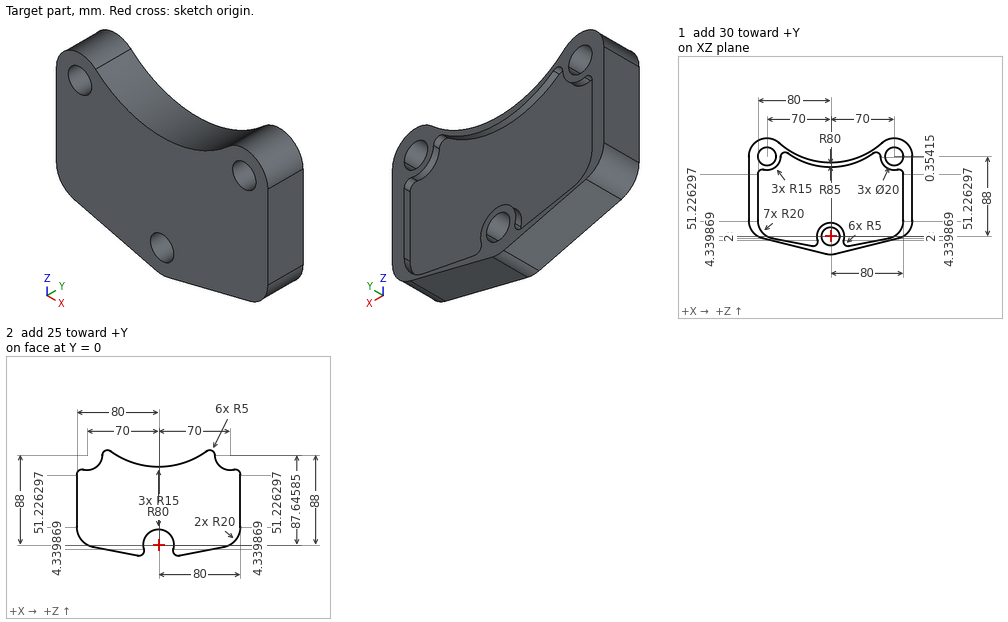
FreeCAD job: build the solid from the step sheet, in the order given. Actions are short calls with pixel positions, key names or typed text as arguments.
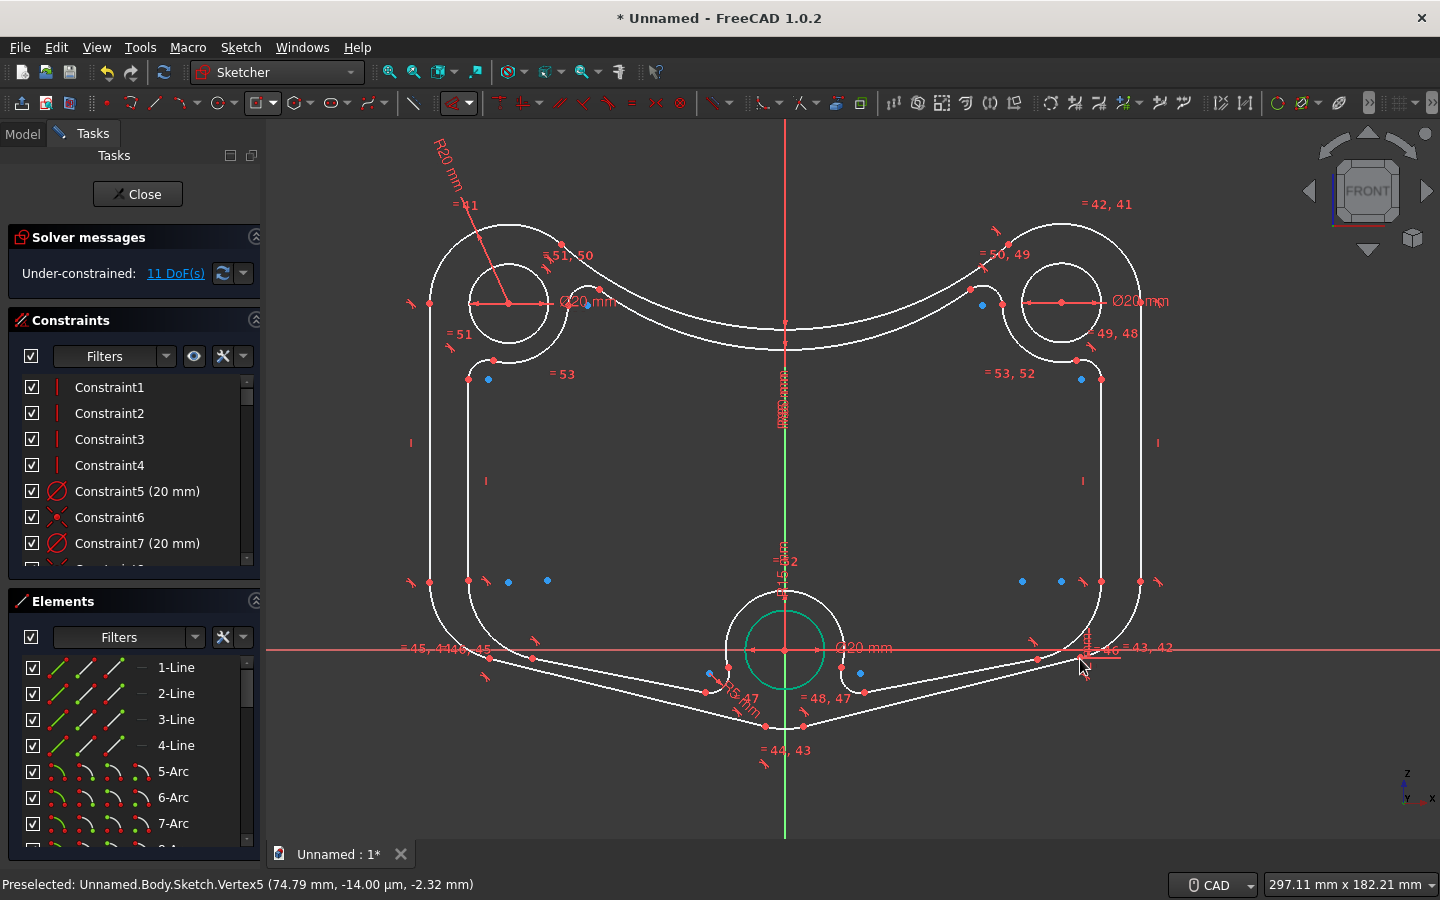
scroll(490, 659, up, 9)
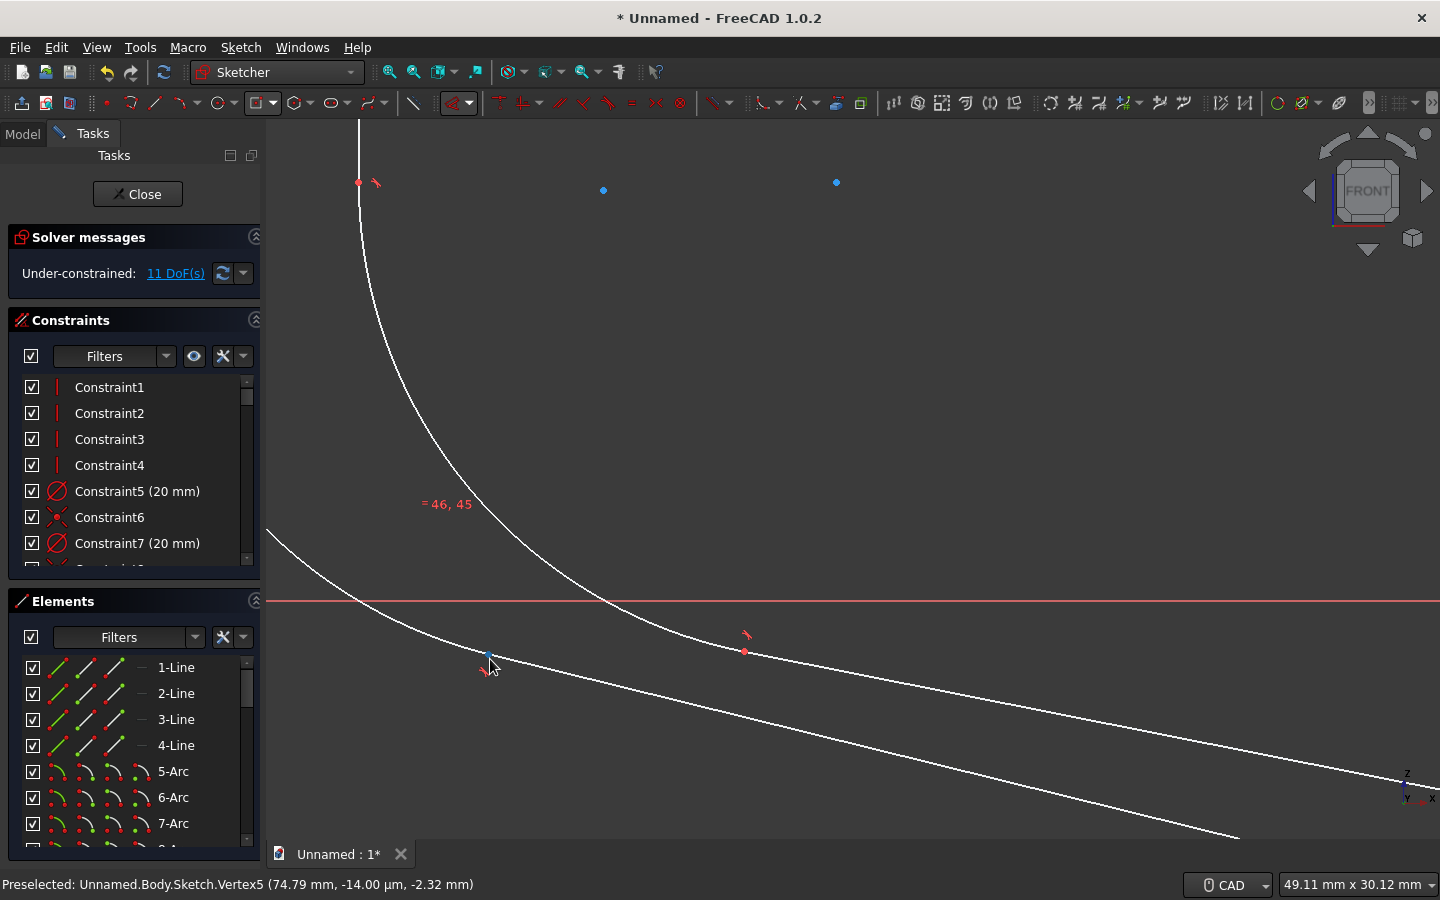
click(489, 654)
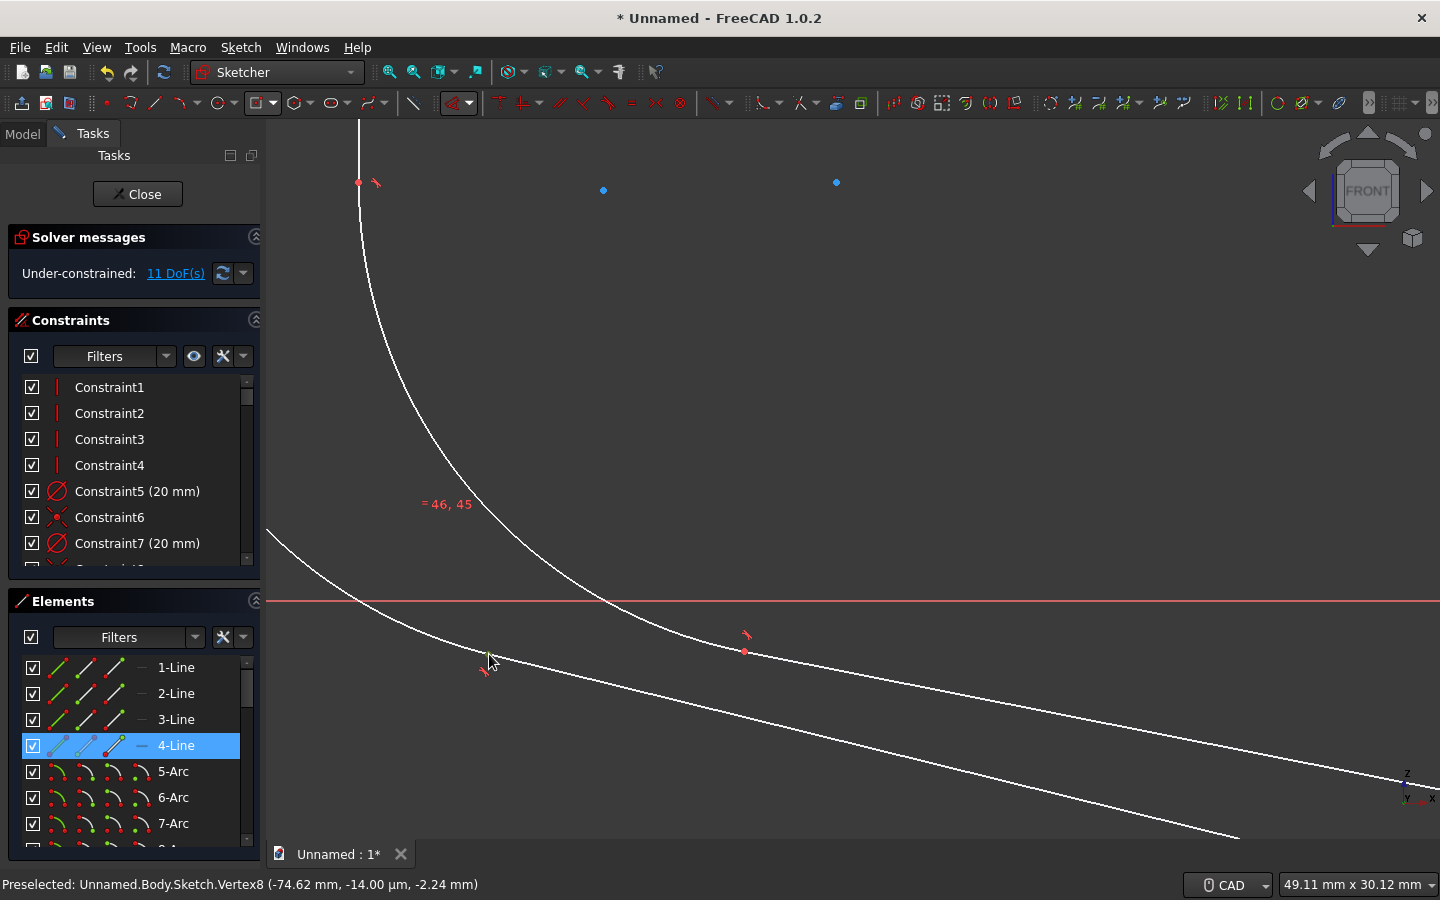
key(i)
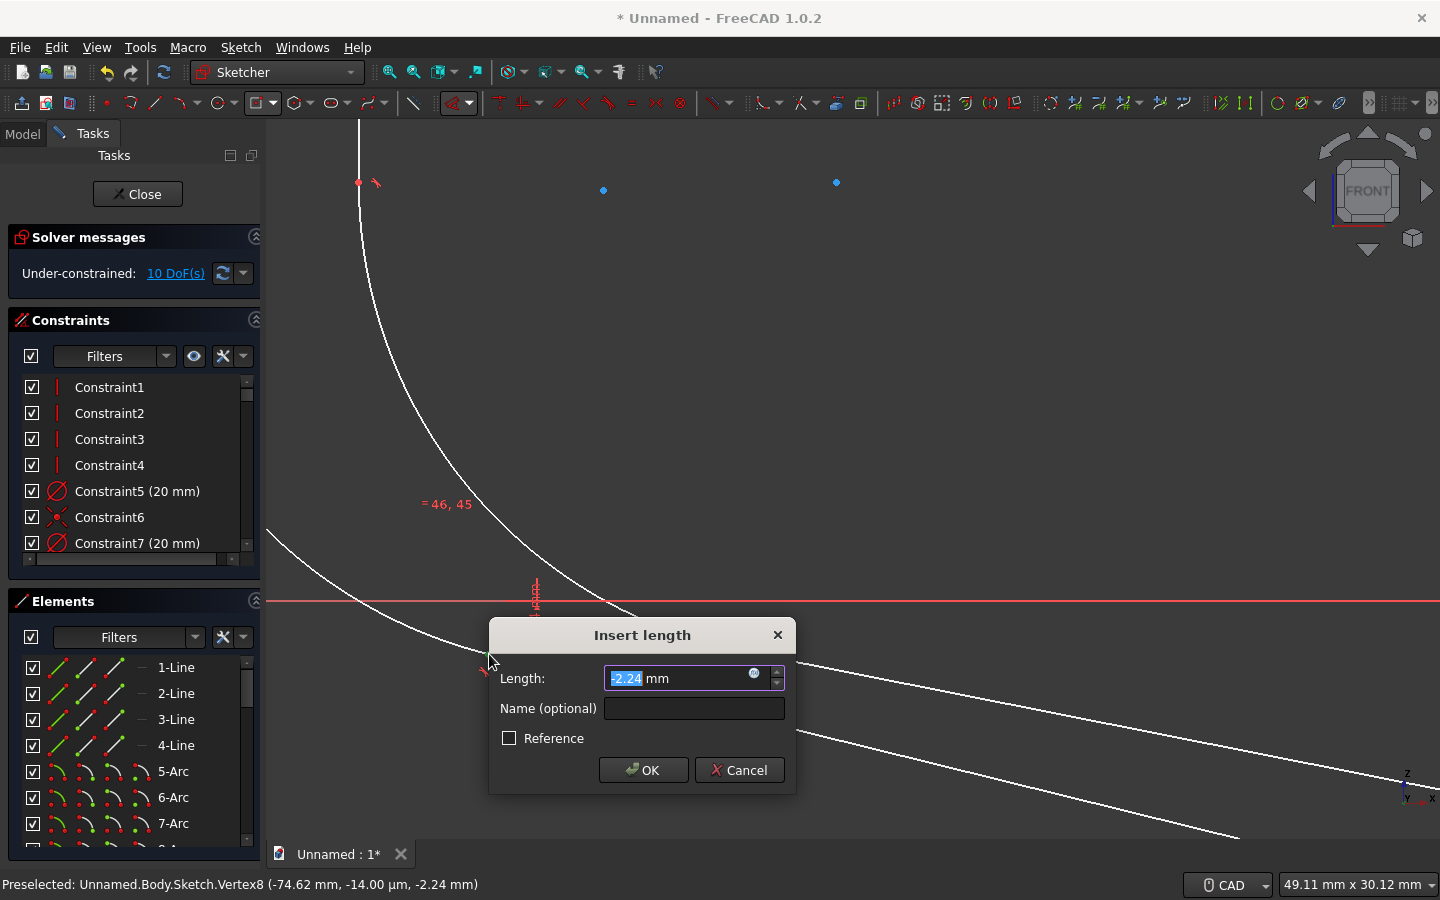
text(-2)
key(Return)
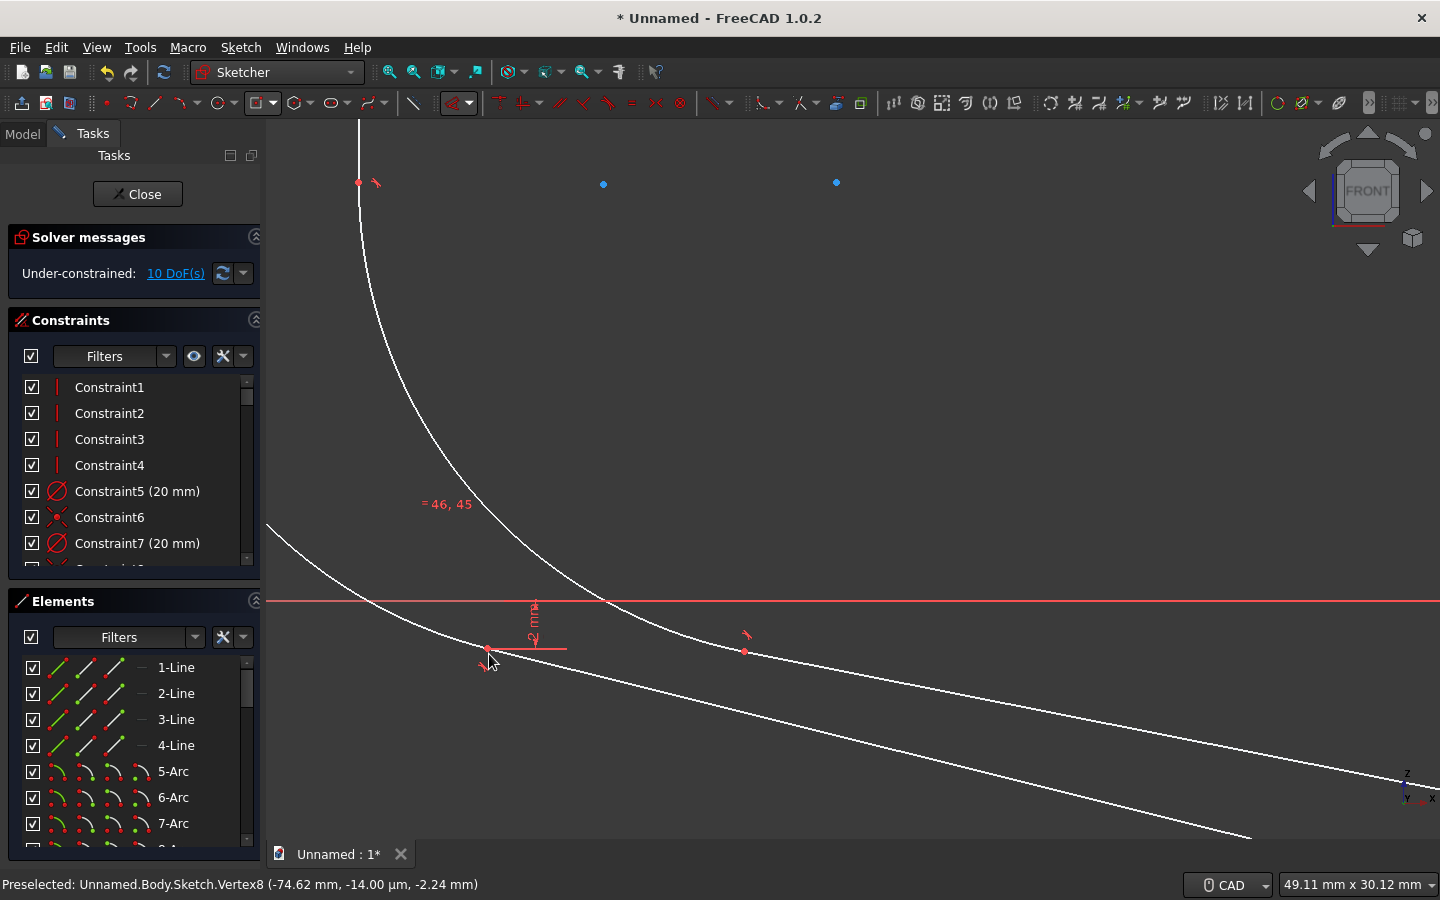
scroll(490, 659, down, 9)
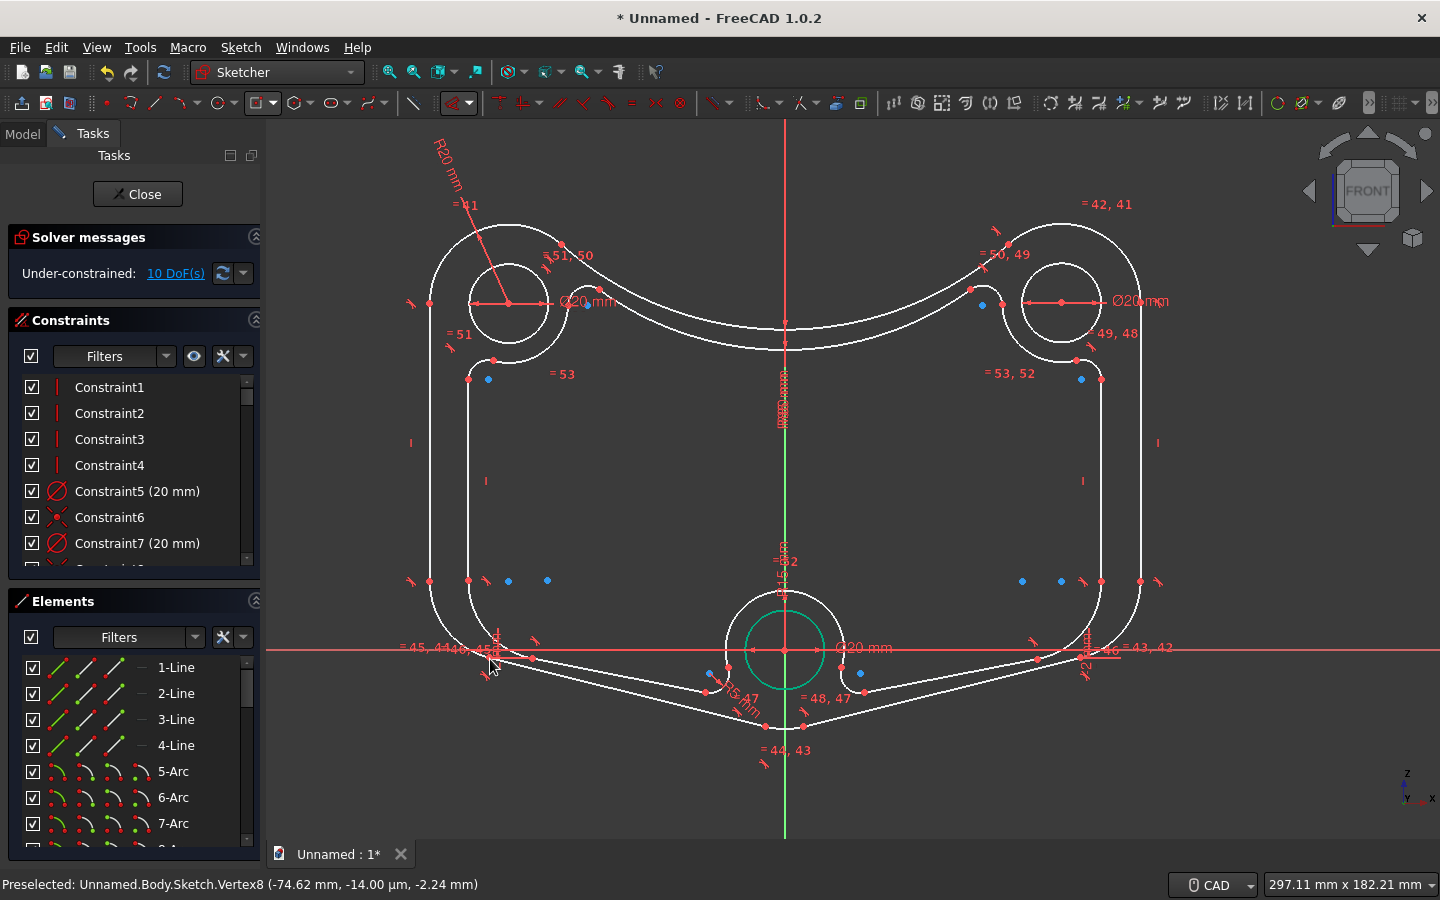
click(1062, 303)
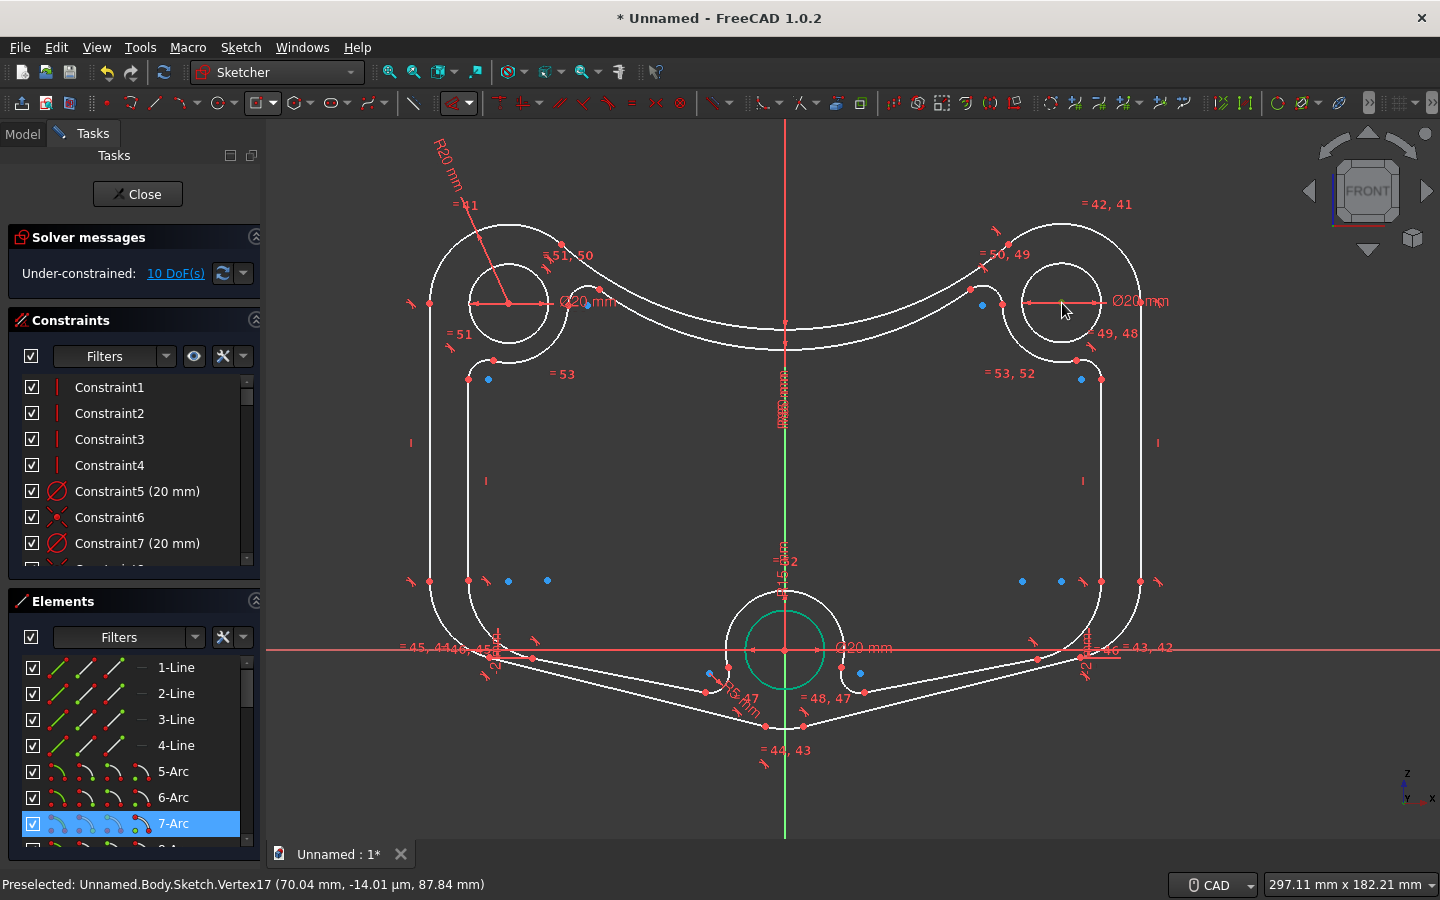
key(l)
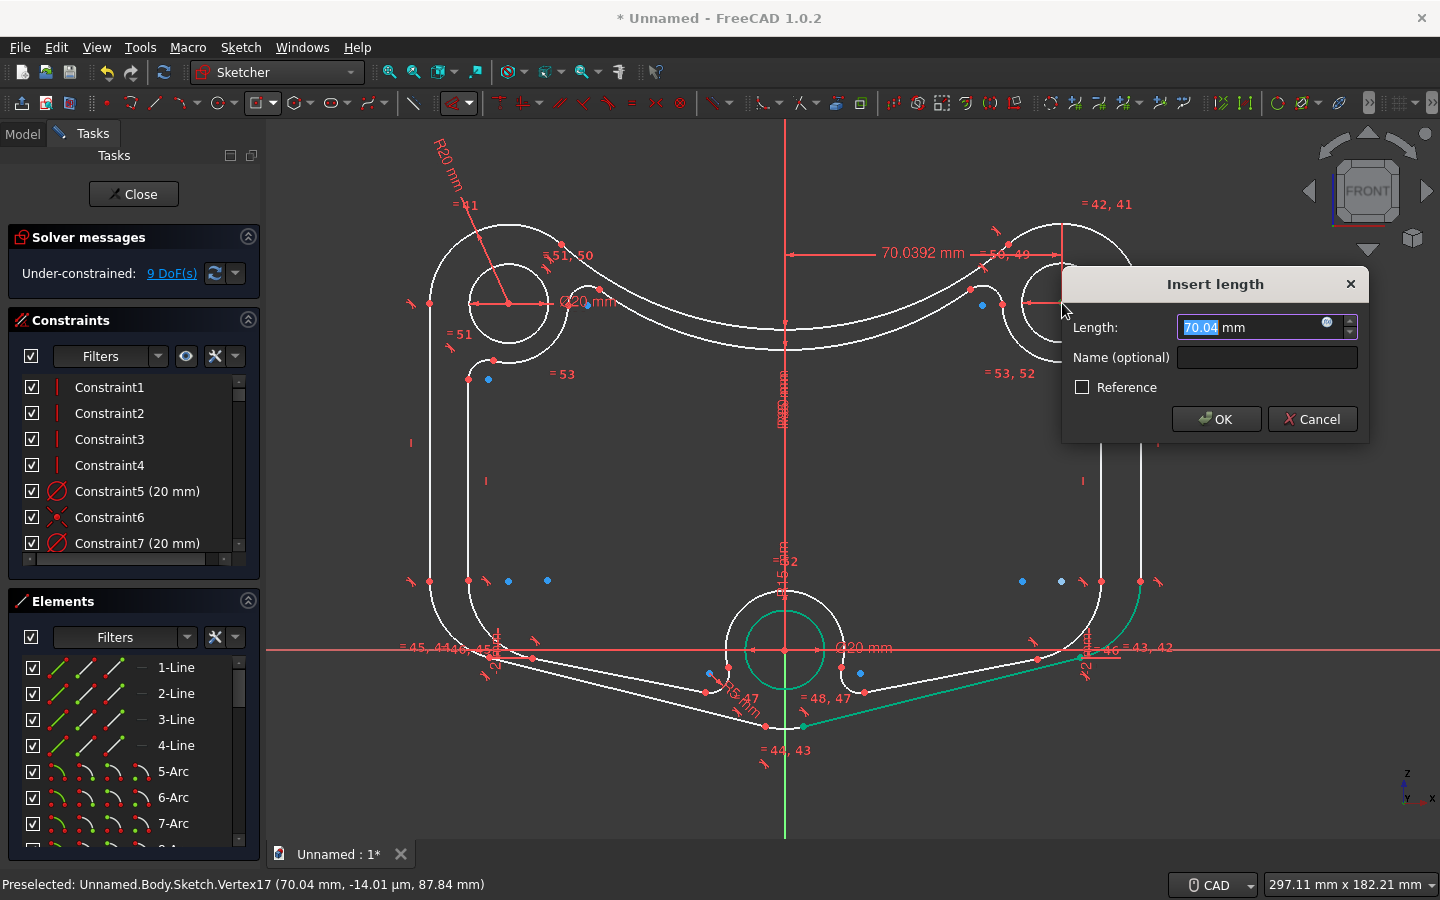
text(70)
key(Return)